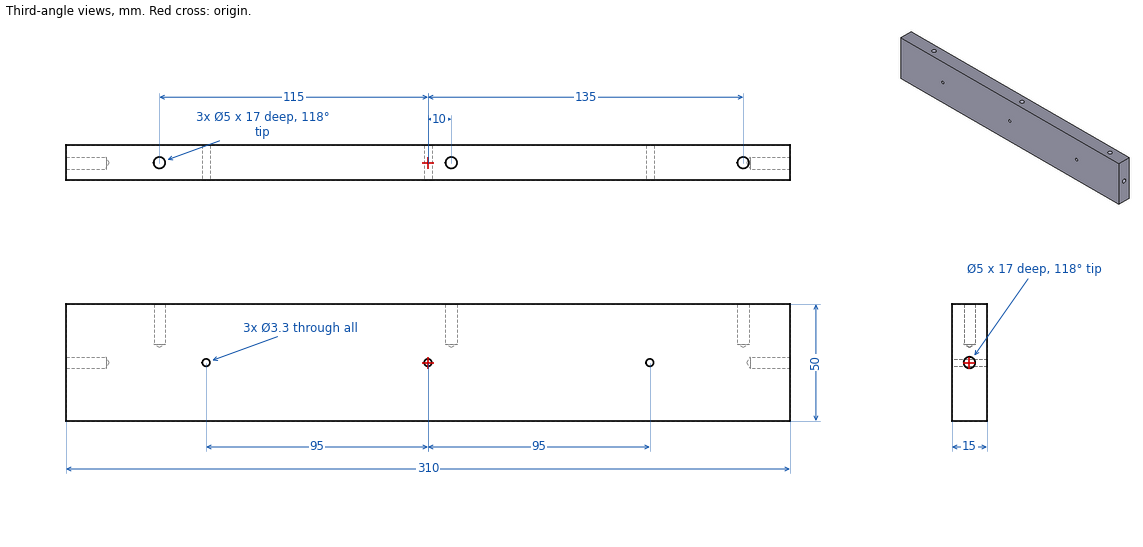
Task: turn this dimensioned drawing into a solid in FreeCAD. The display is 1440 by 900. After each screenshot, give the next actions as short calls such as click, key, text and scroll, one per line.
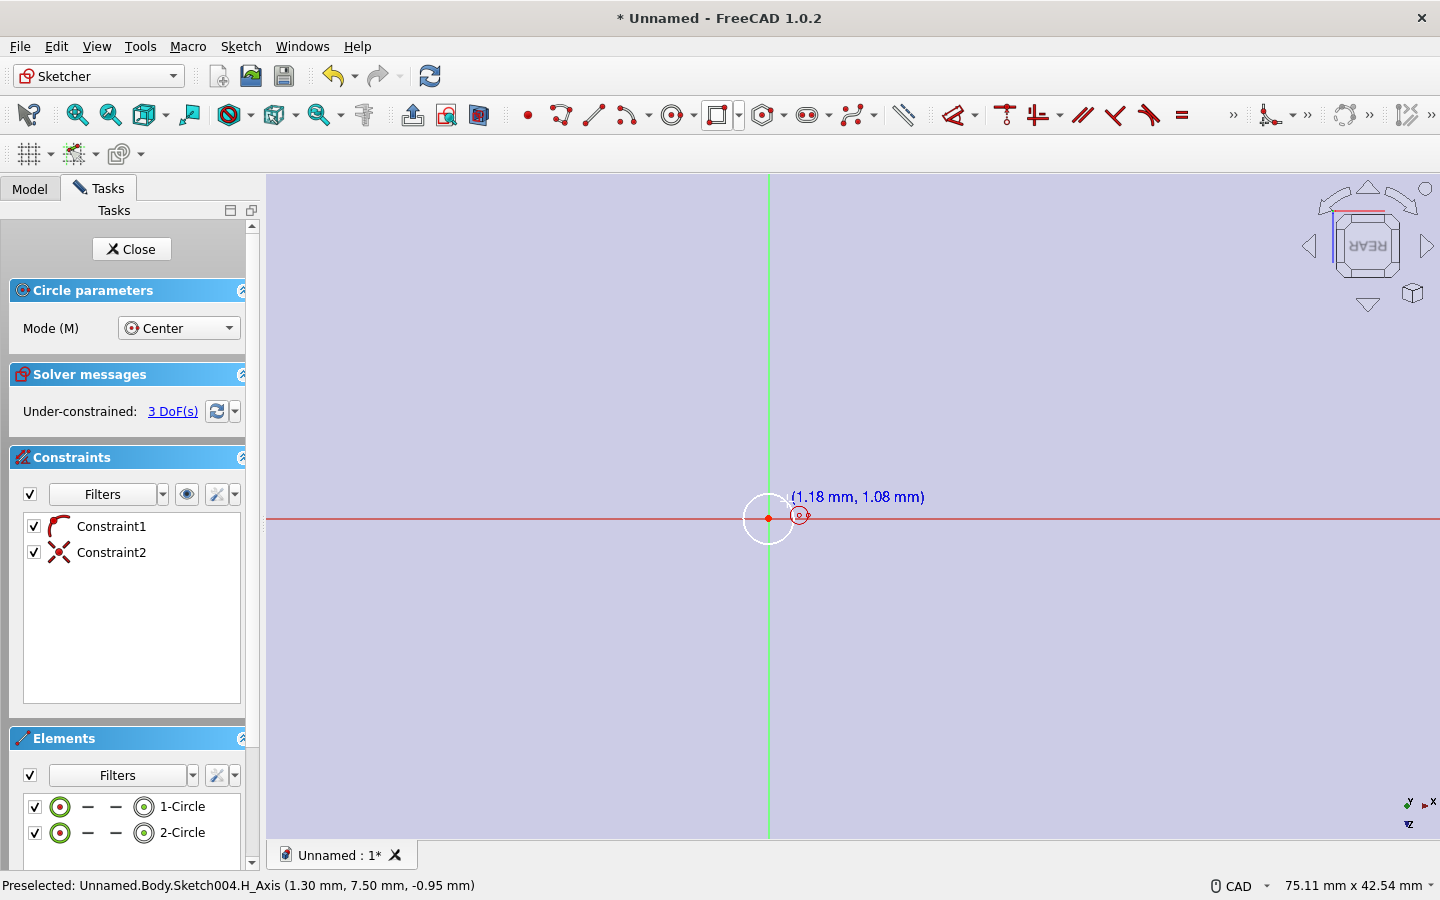
scroll(790, 502, down, 7)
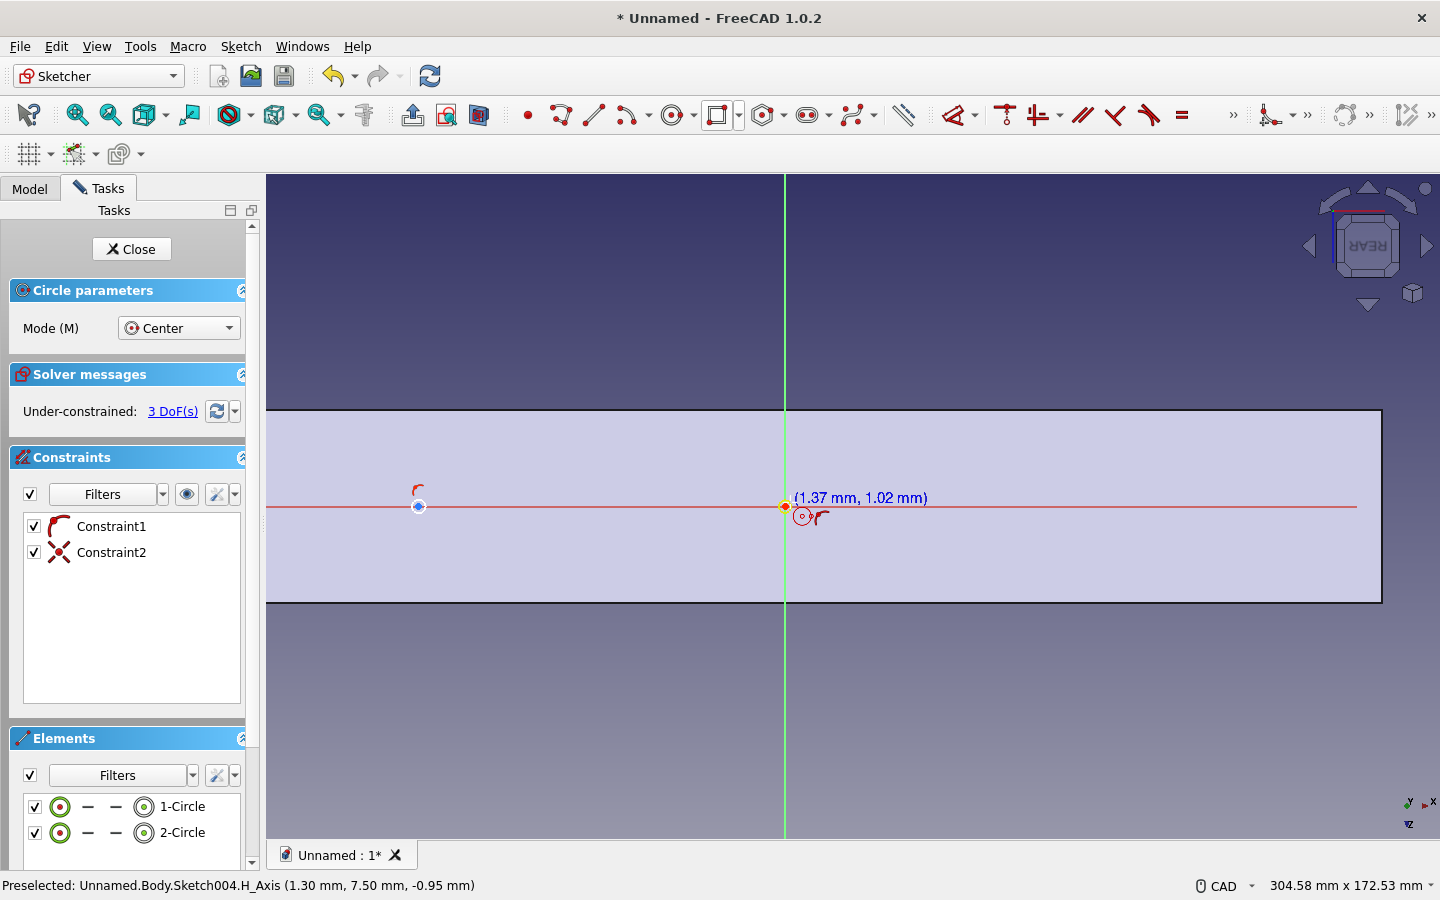
scroll(1151, 507, up, 7)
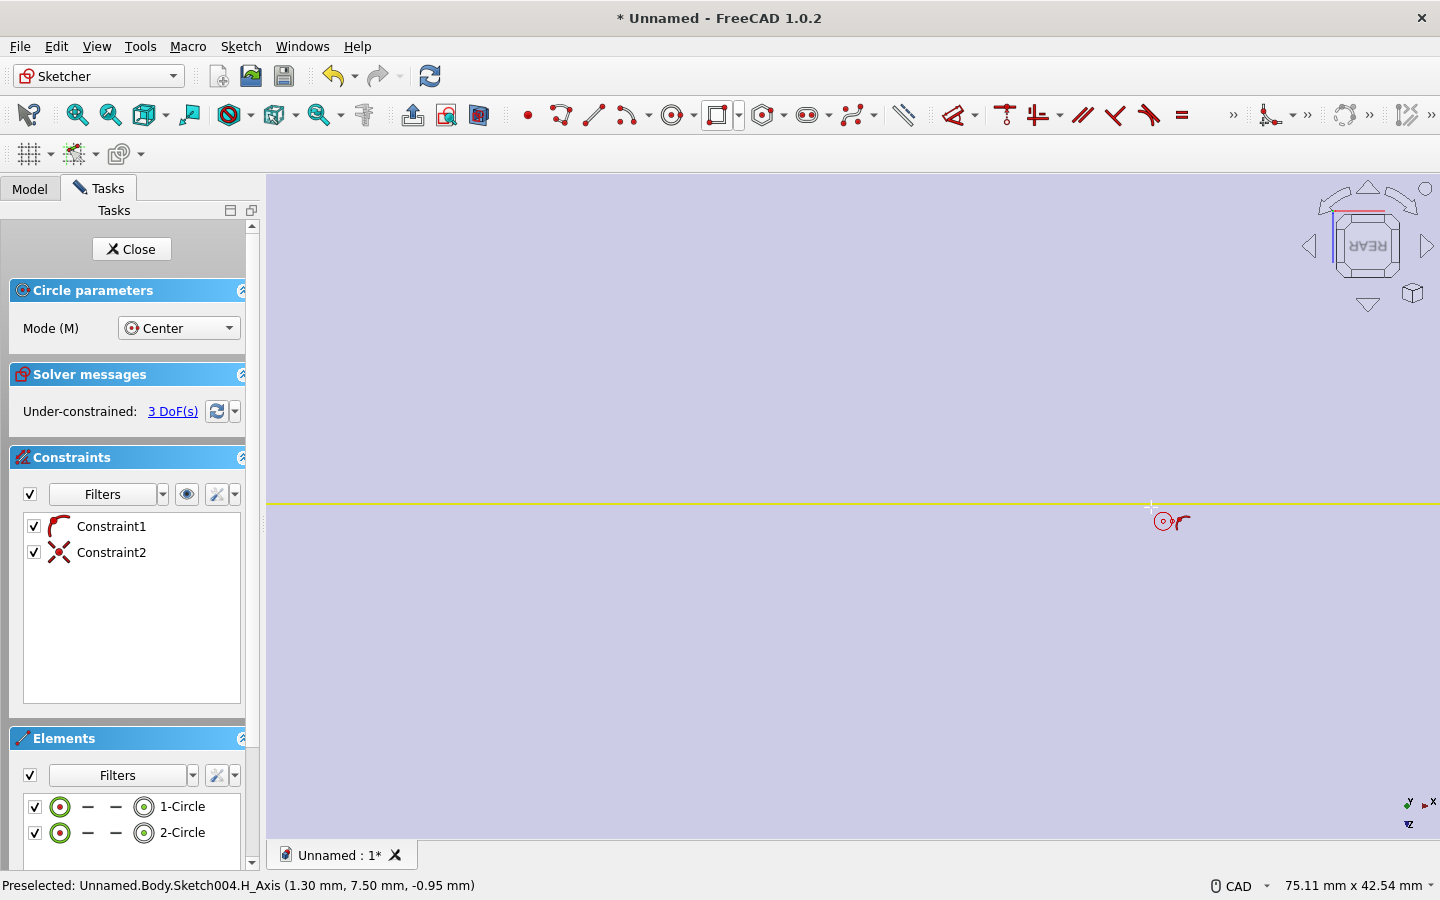
scroll(1151, 507, down, 7)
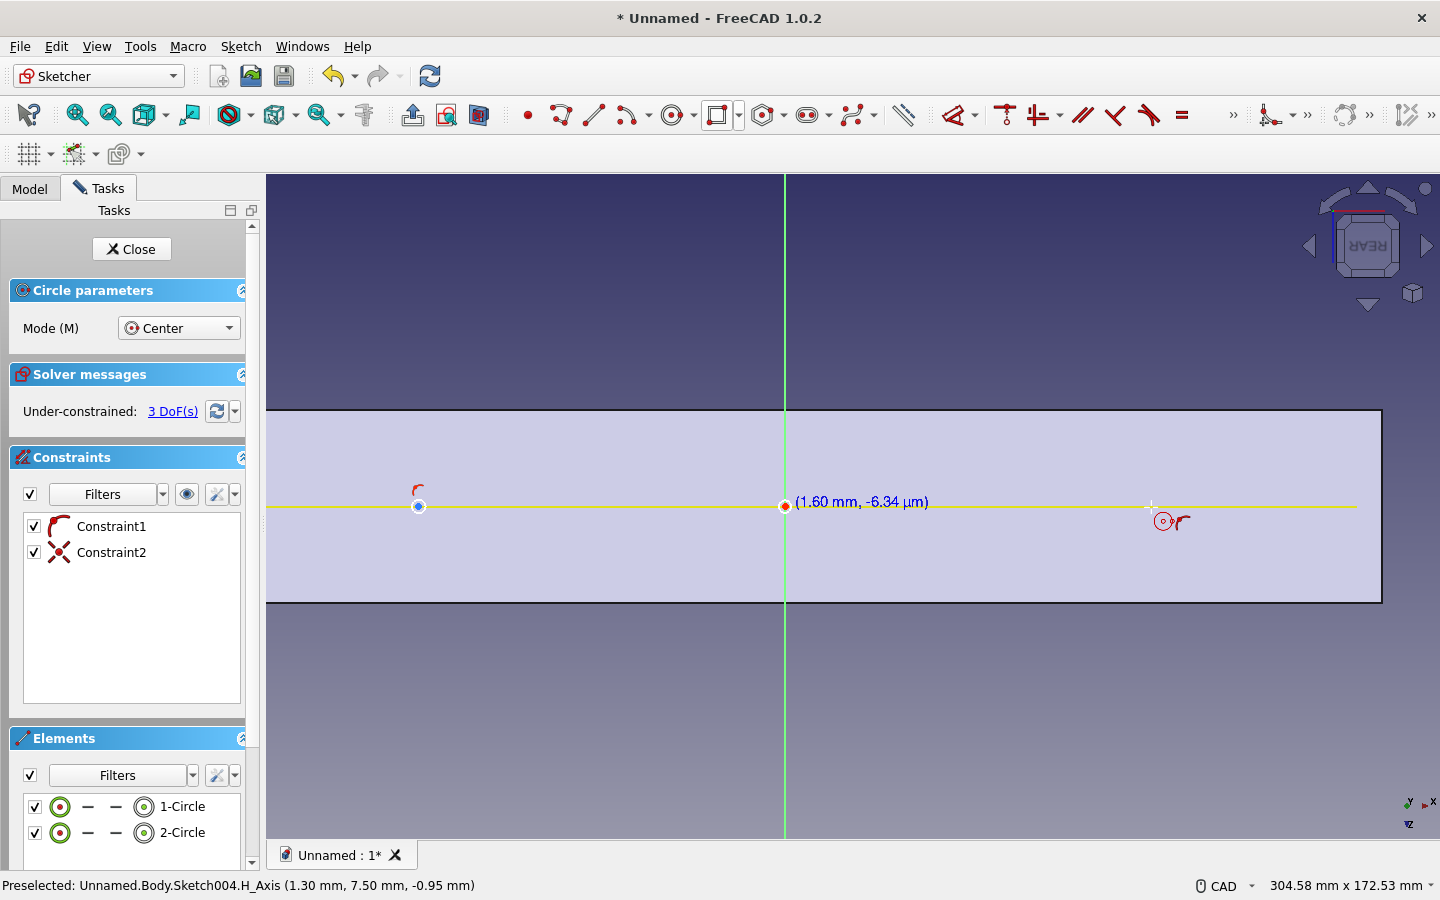
click(1151, 507)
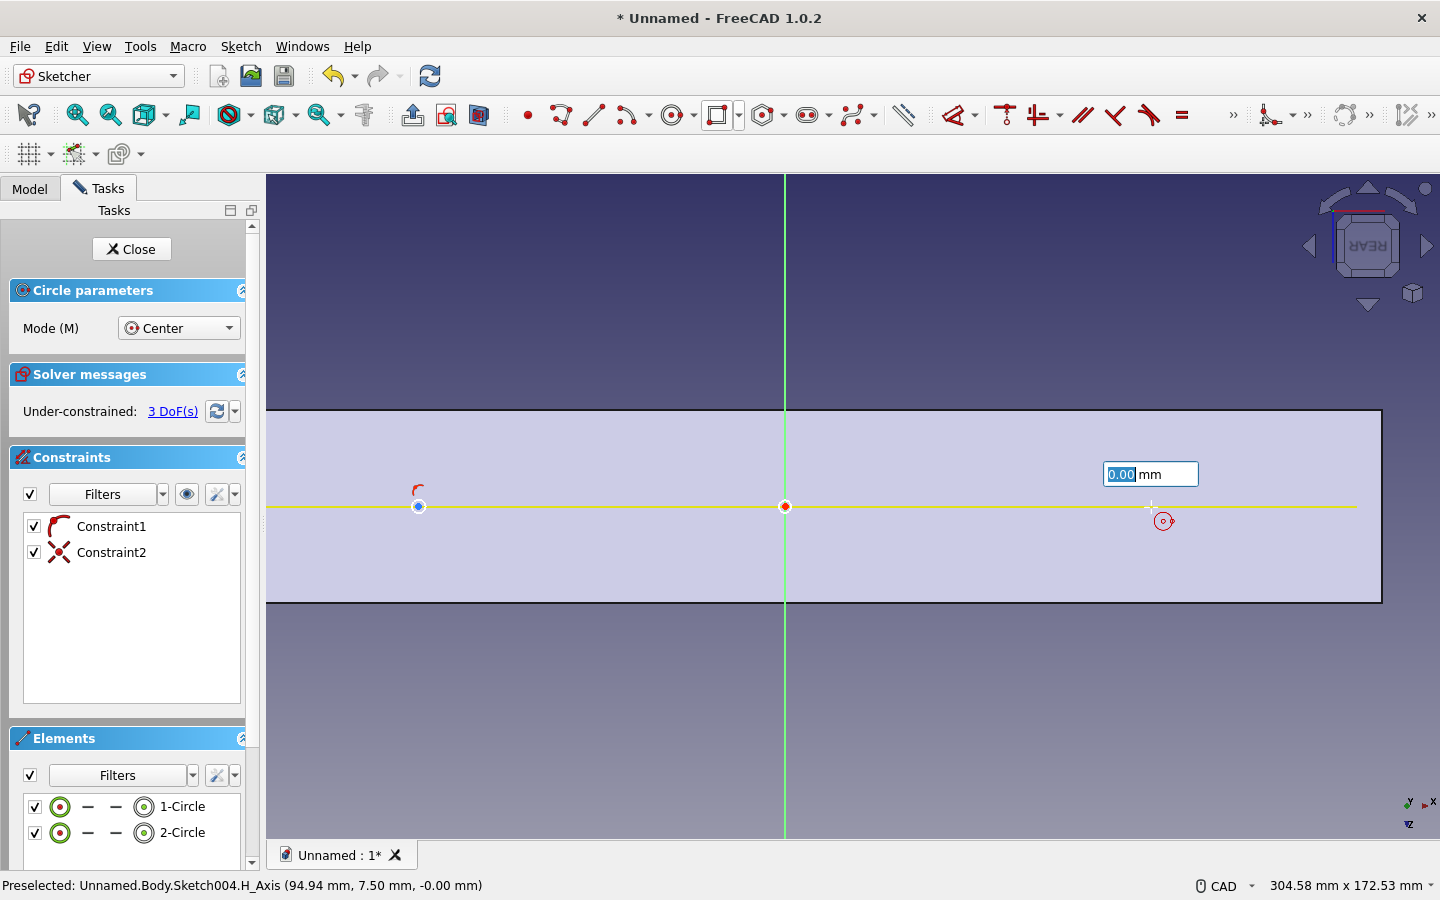
scroll(1149, 513, up, 5)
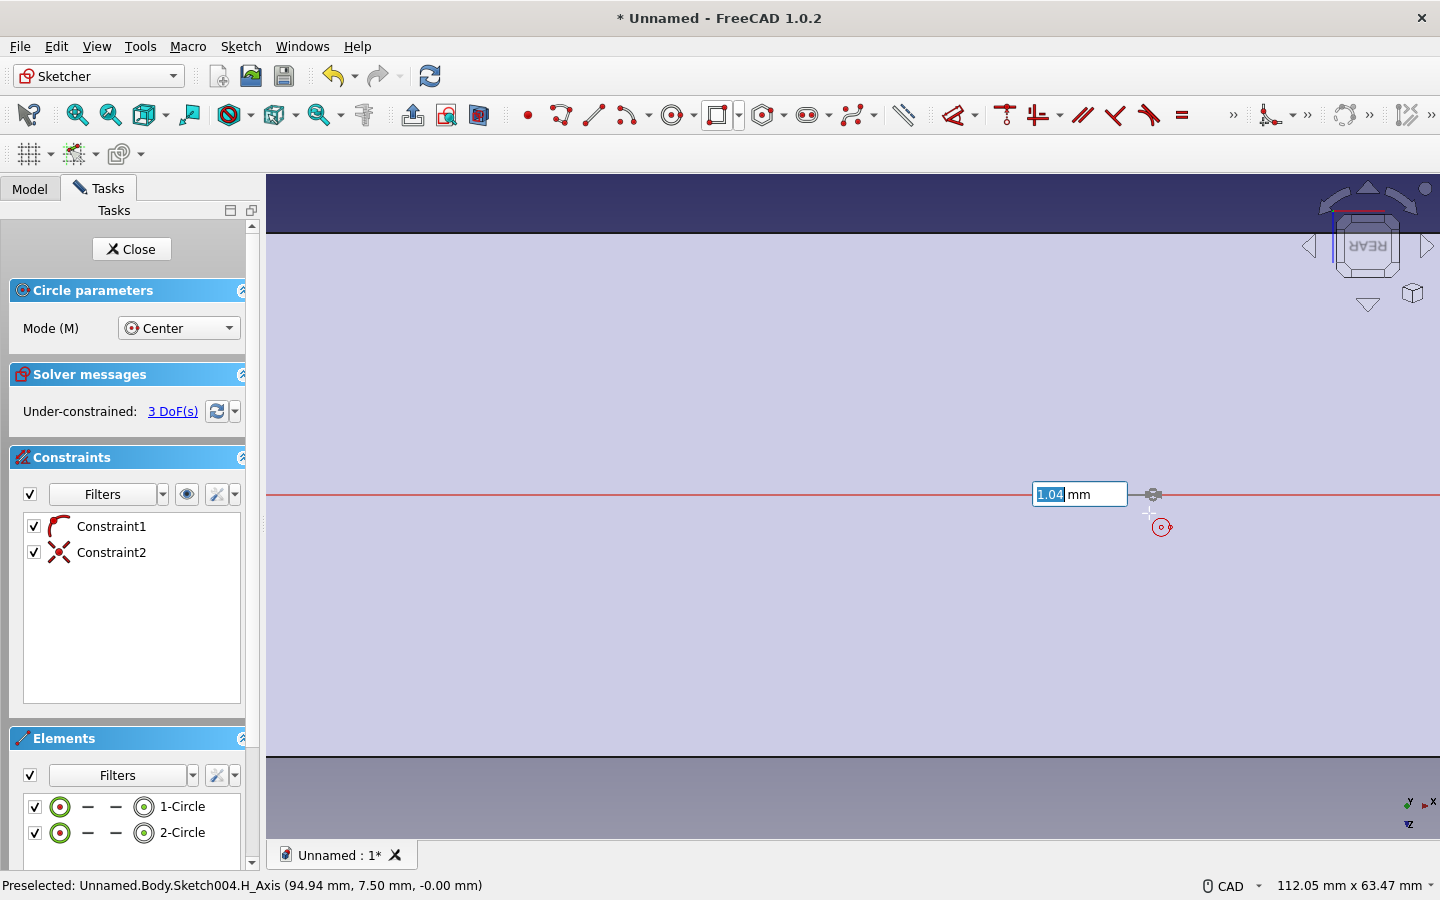
click(1148, 511)
key(Escape)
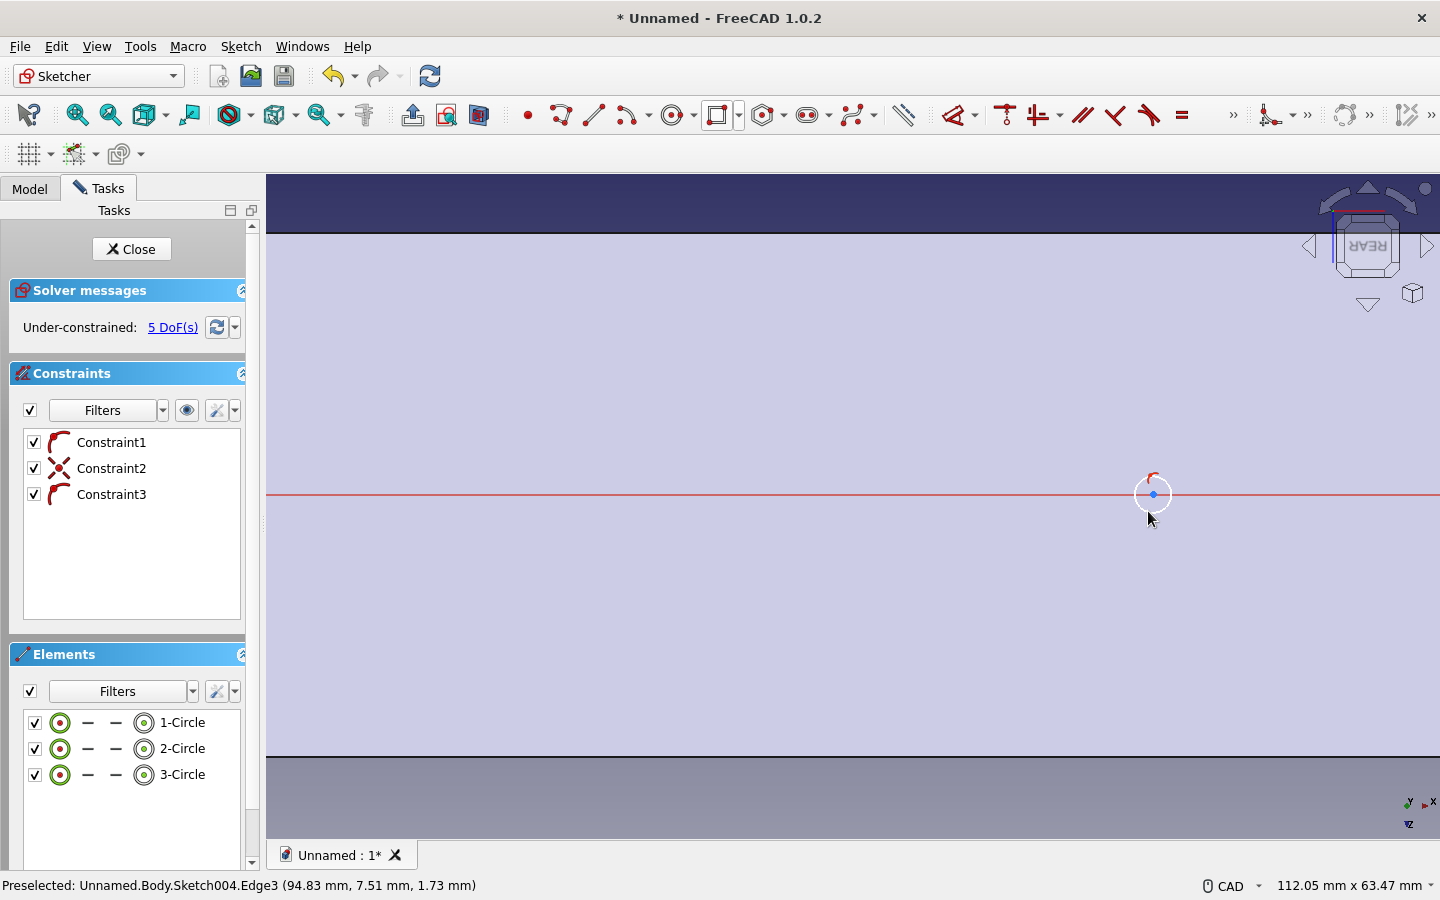
scroll(1149, 513, down, 5)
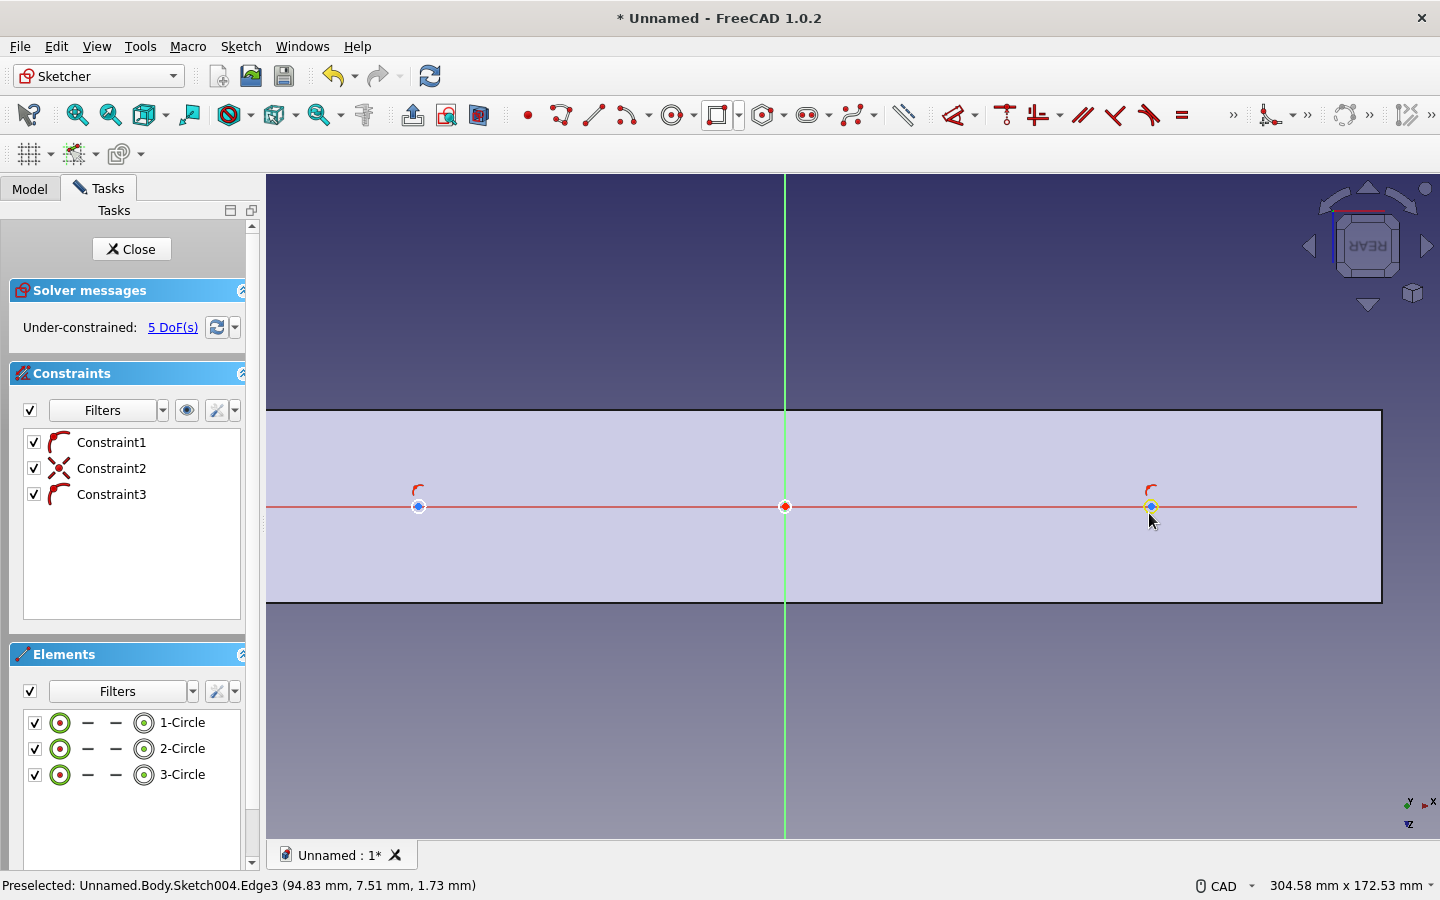
scroll(424, 502, up, 6)